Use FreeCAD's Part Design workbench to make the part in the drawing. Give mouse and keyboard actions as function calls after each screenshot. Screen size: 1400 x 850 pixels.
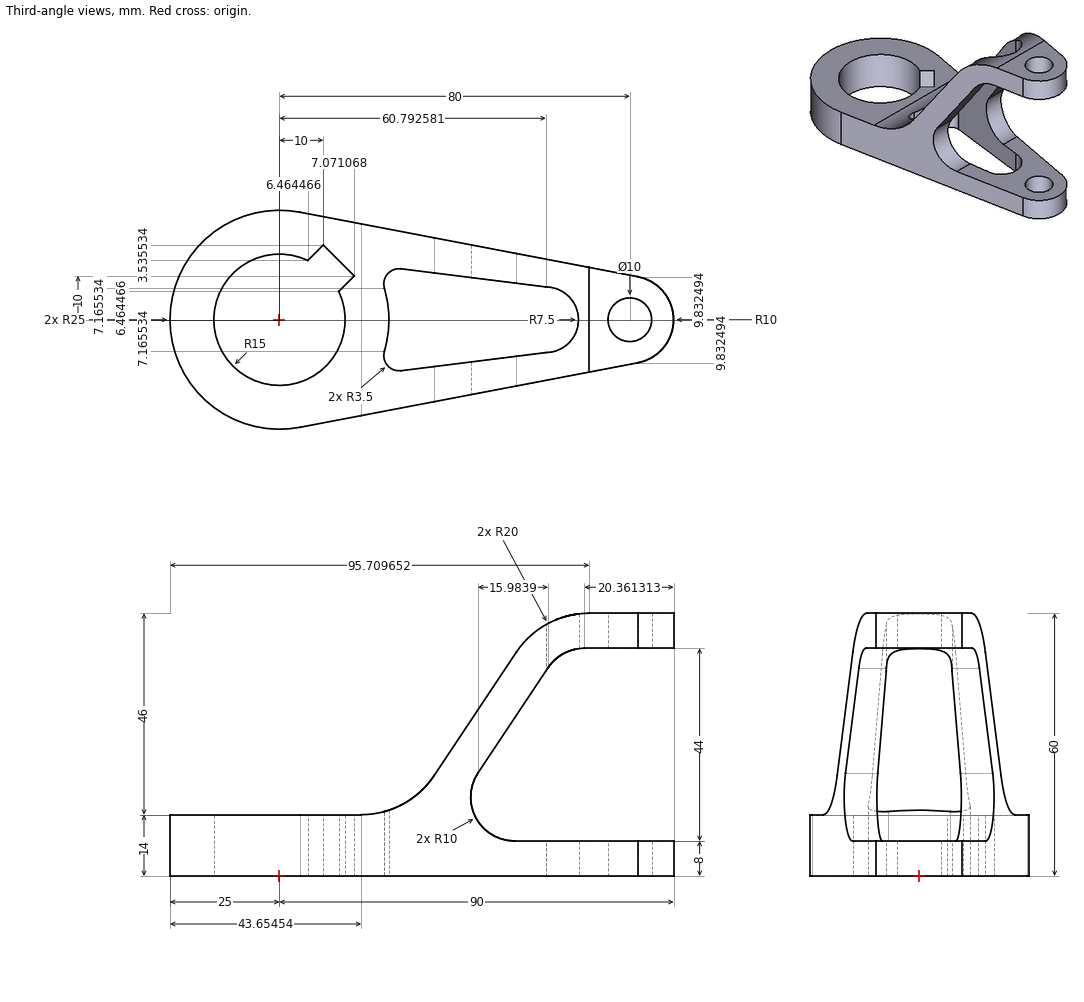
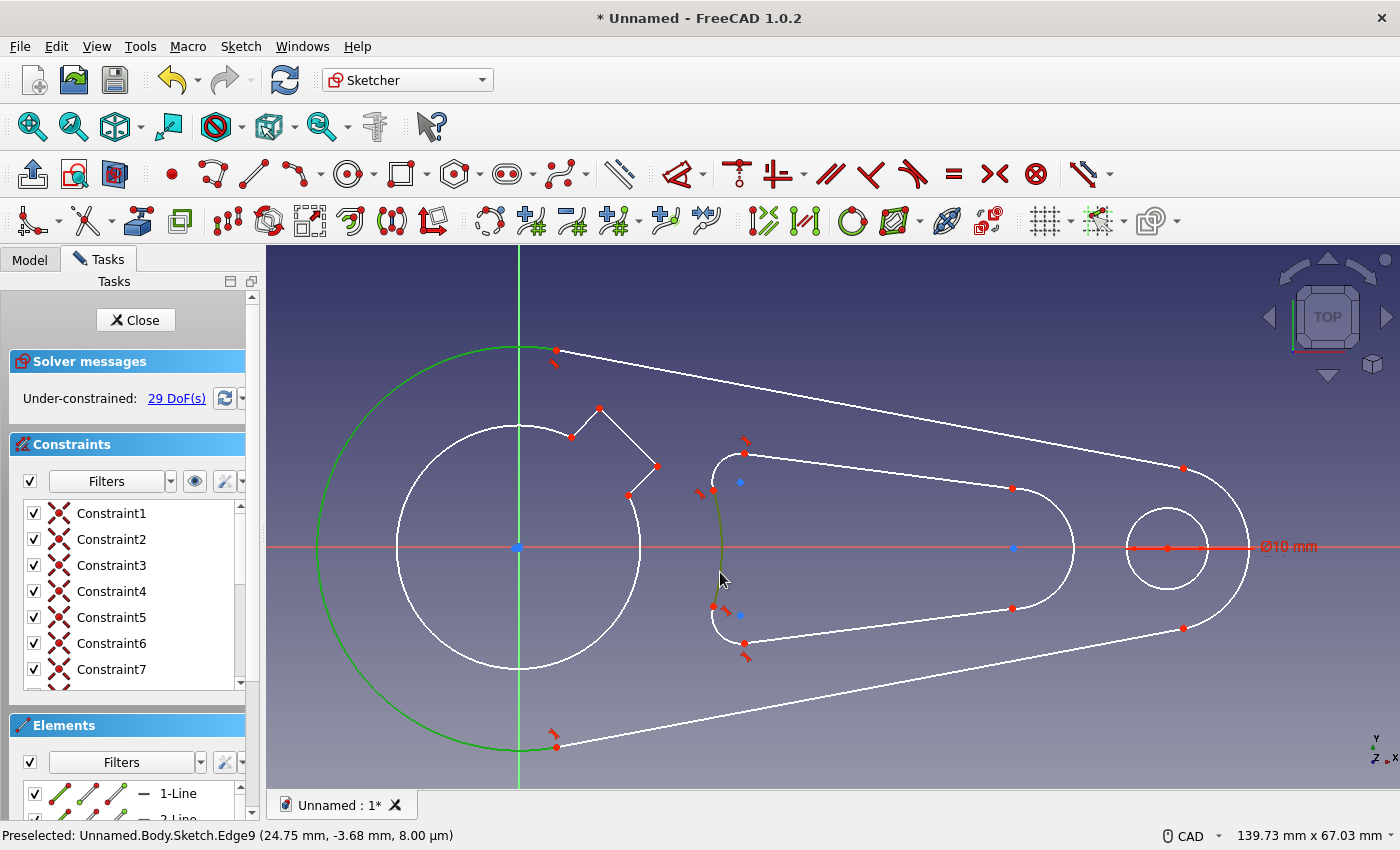
key(c)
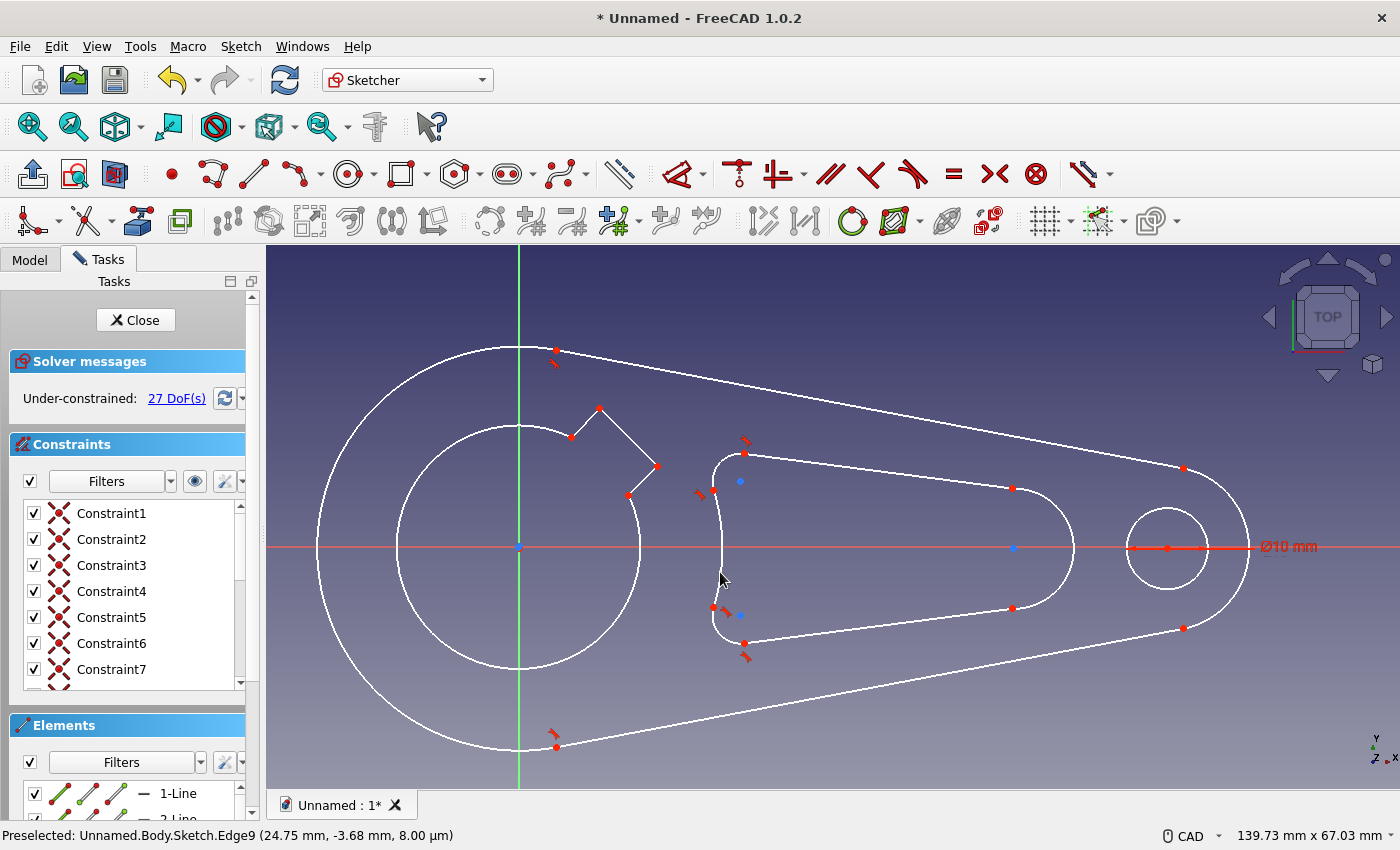
click(365, 418)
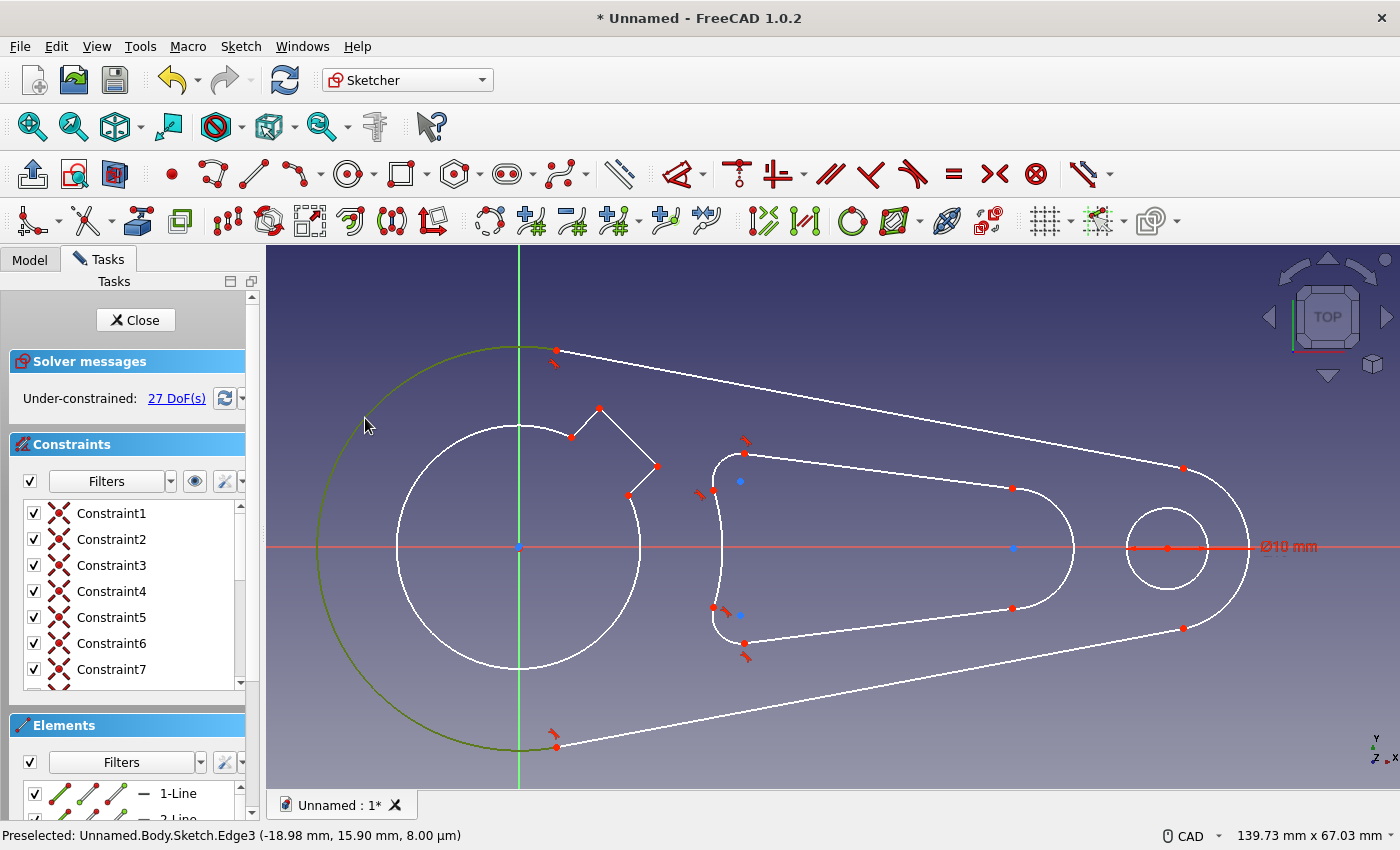
click(404, 506)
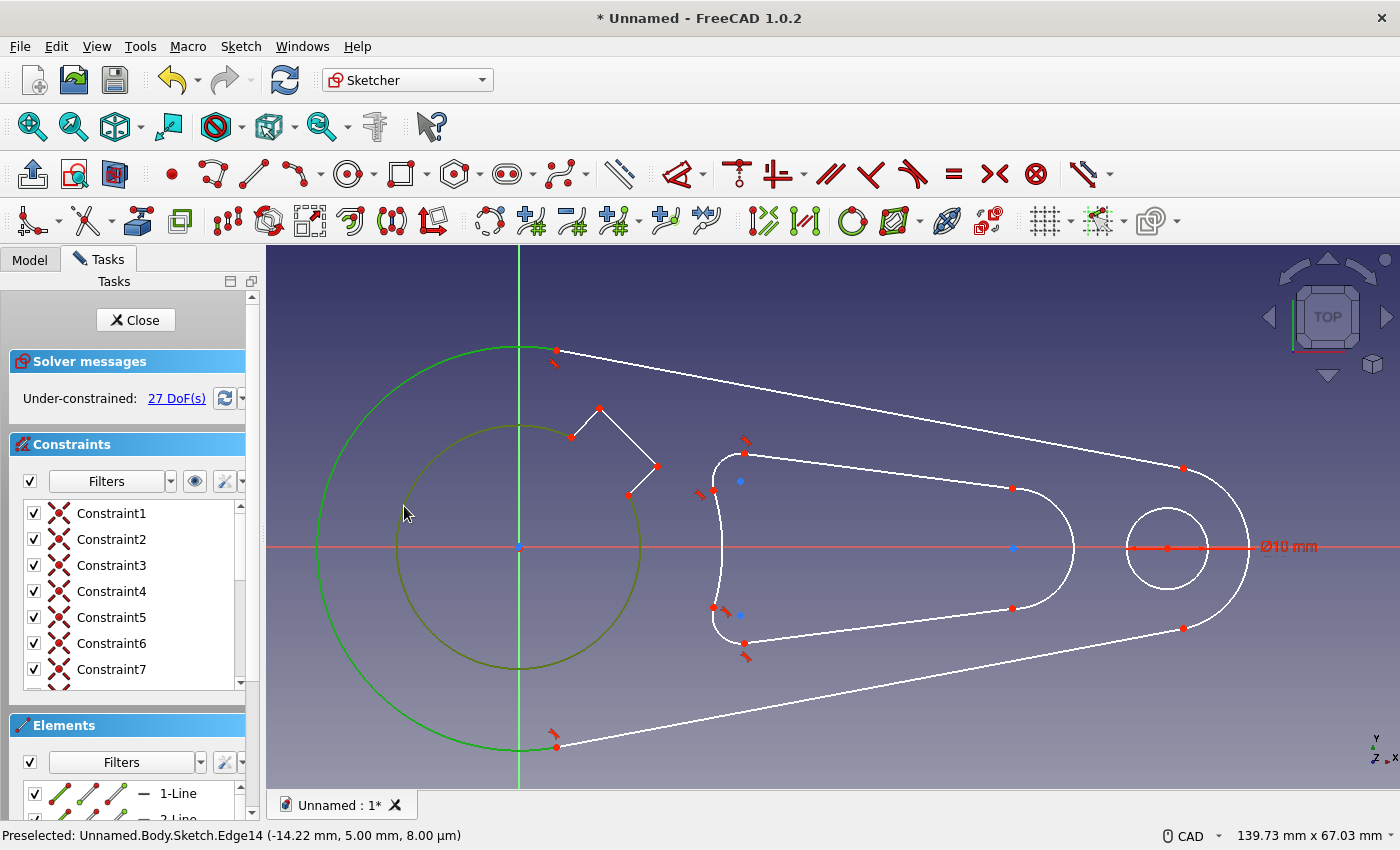
click(737, 174)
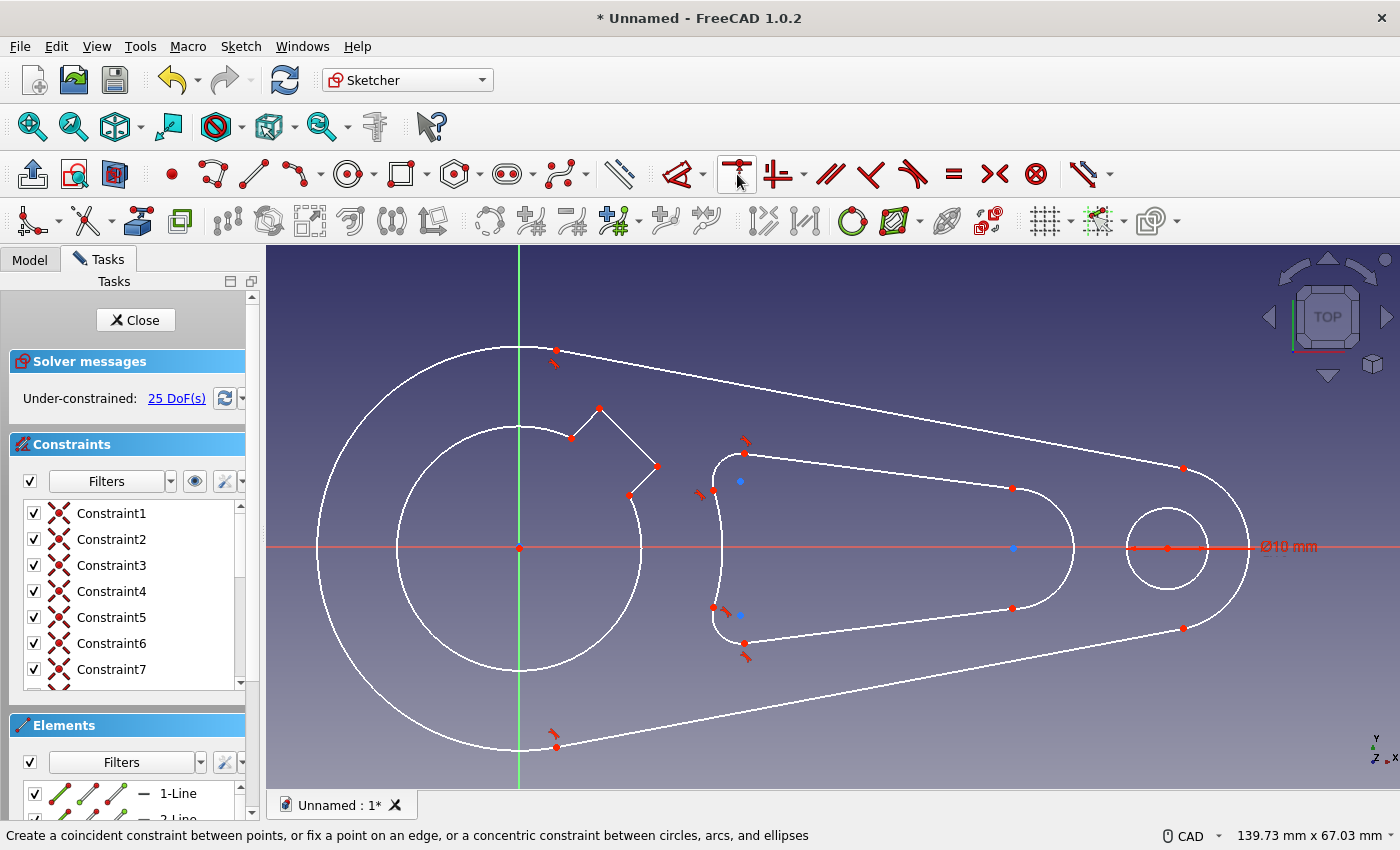
scroll(519, 548, up, 2)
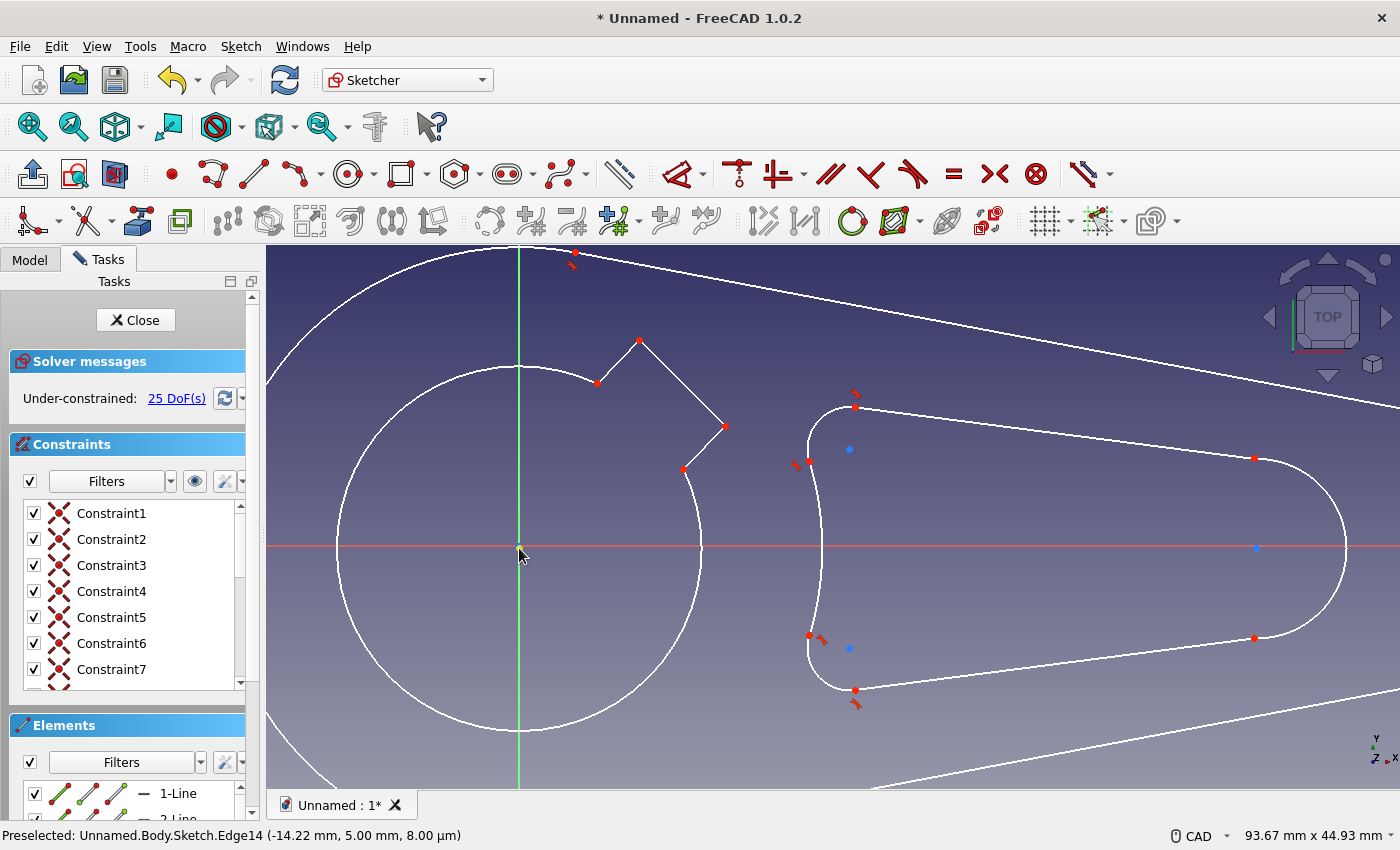
drag(509, 536, 529, 559)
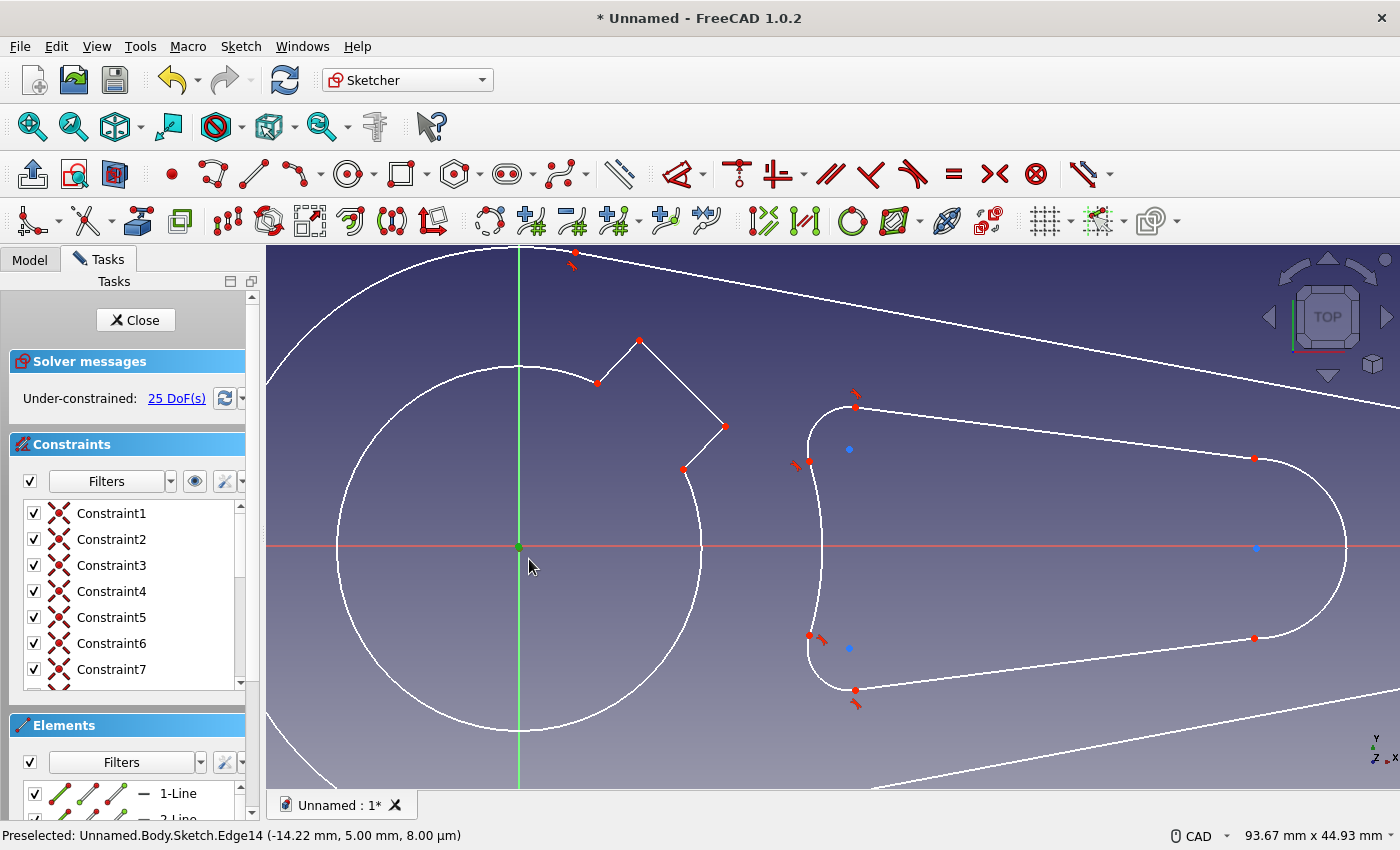
click(737, 174)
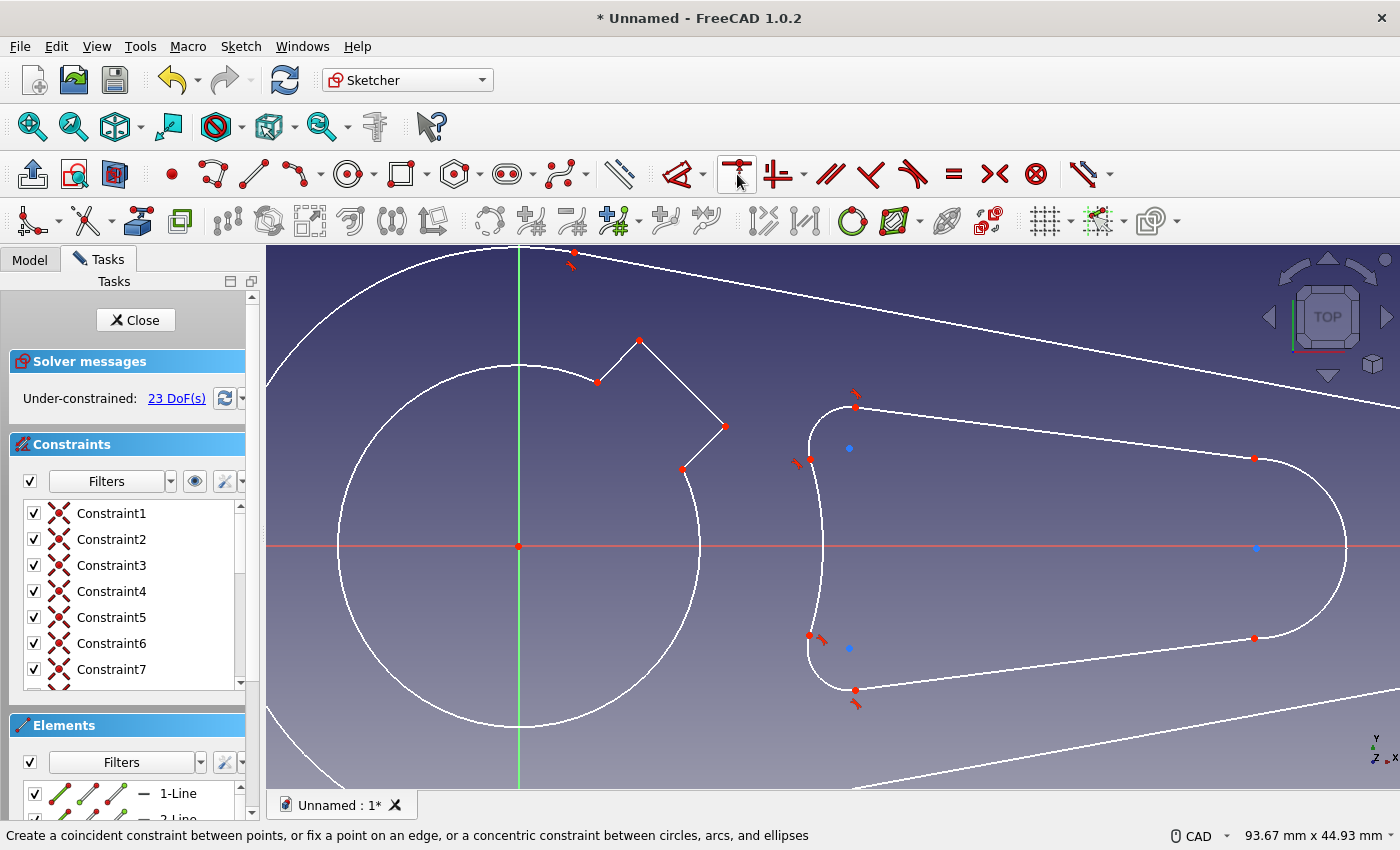
click(372, 286)